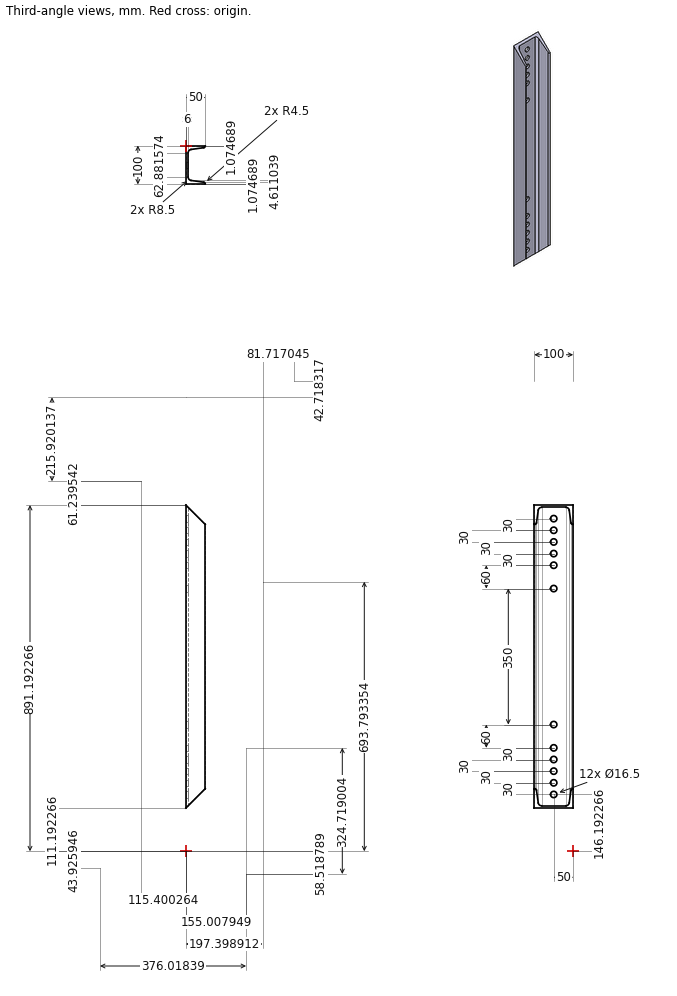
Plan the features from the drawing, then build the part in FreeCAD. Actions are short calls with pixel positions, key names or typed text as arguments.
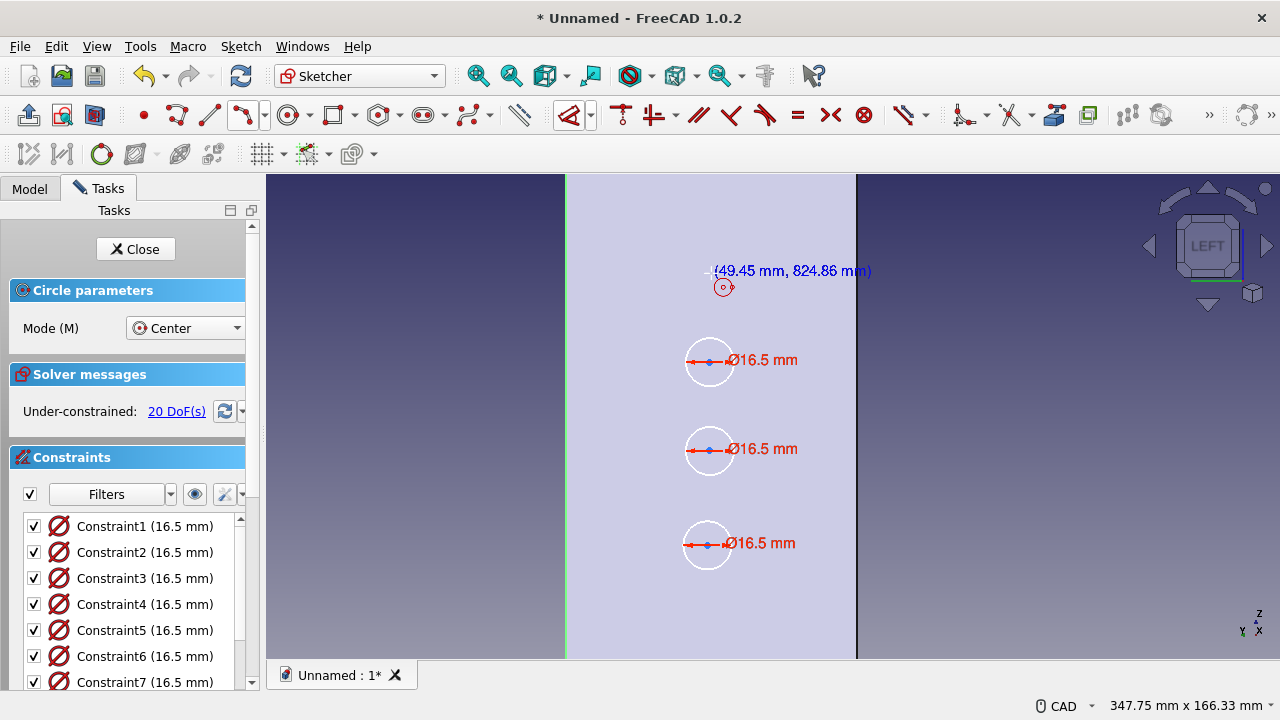
scroll(711, 291, down, 11)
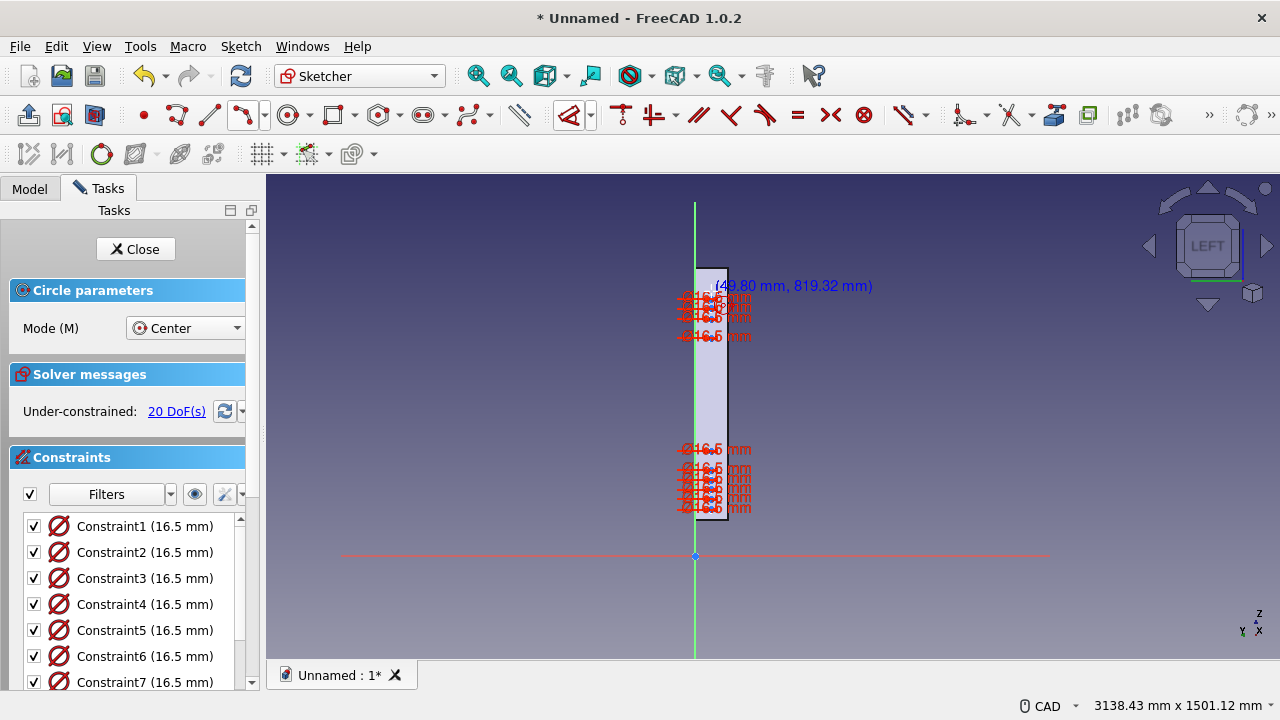
scroll(711, 289, up, 5)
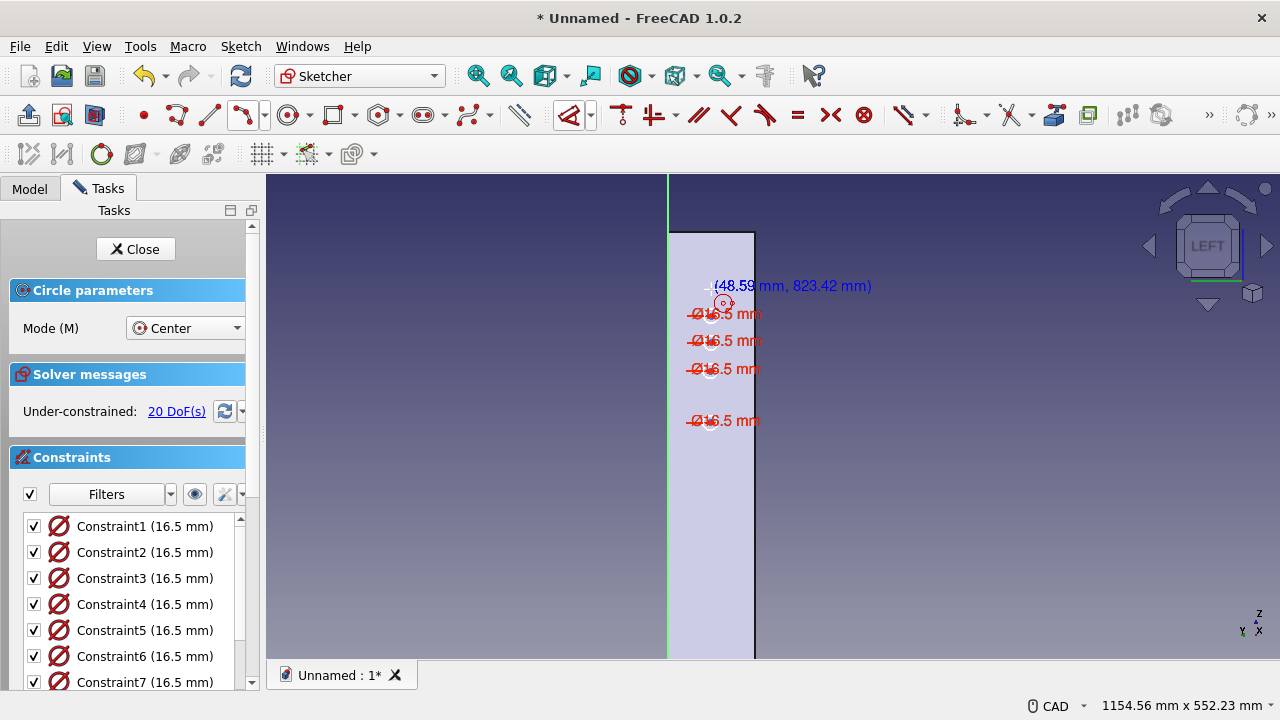
click(711, 289)
move(717, 284)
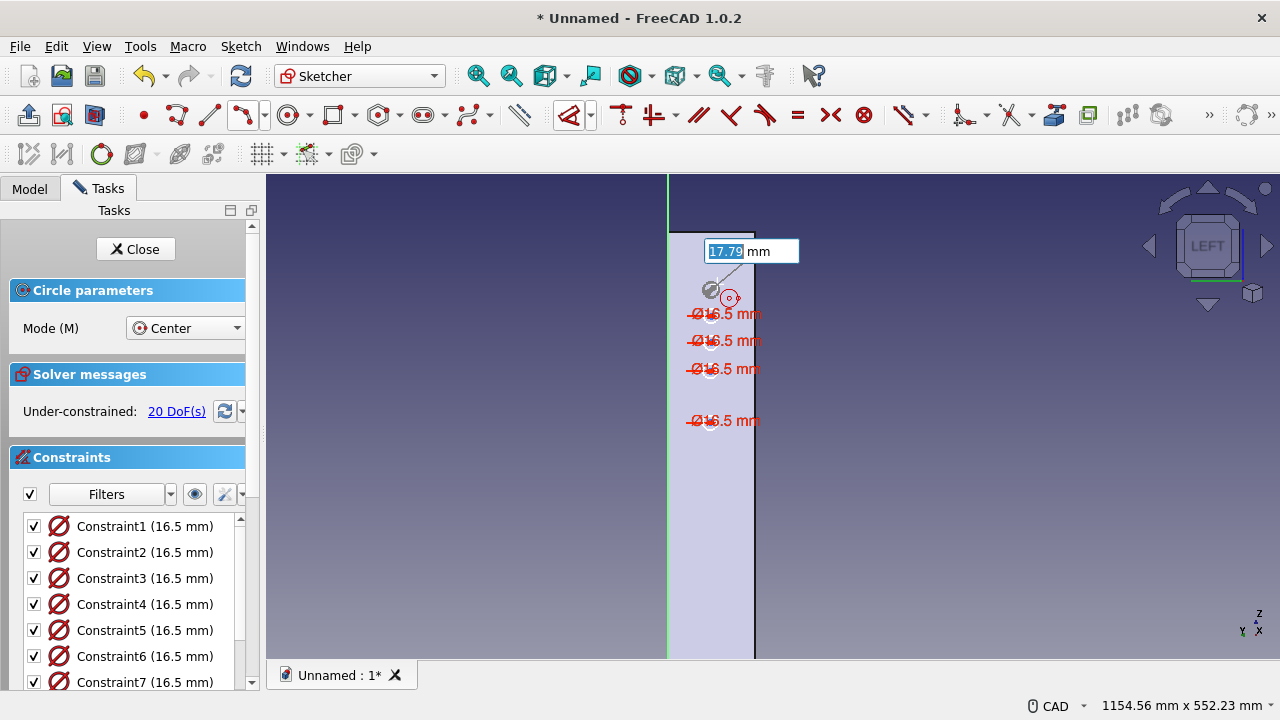
text(16.5)
key(Return)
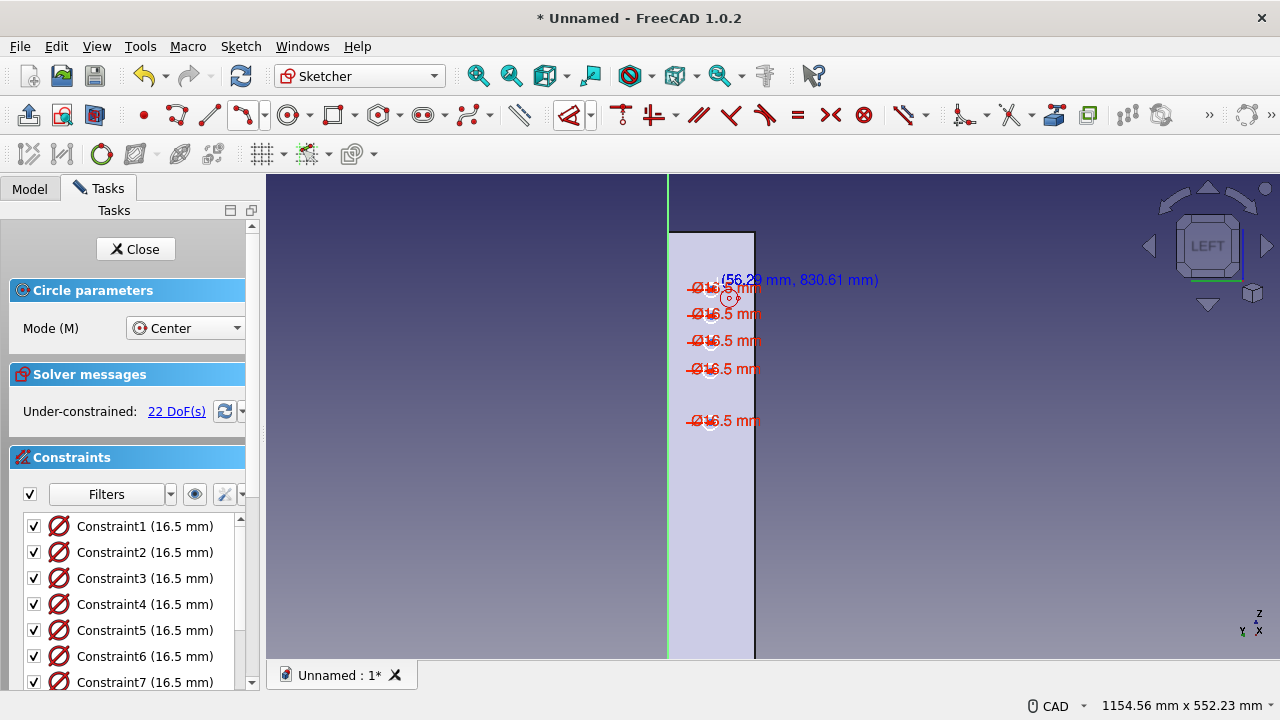
scroll(711, 263, up, 6)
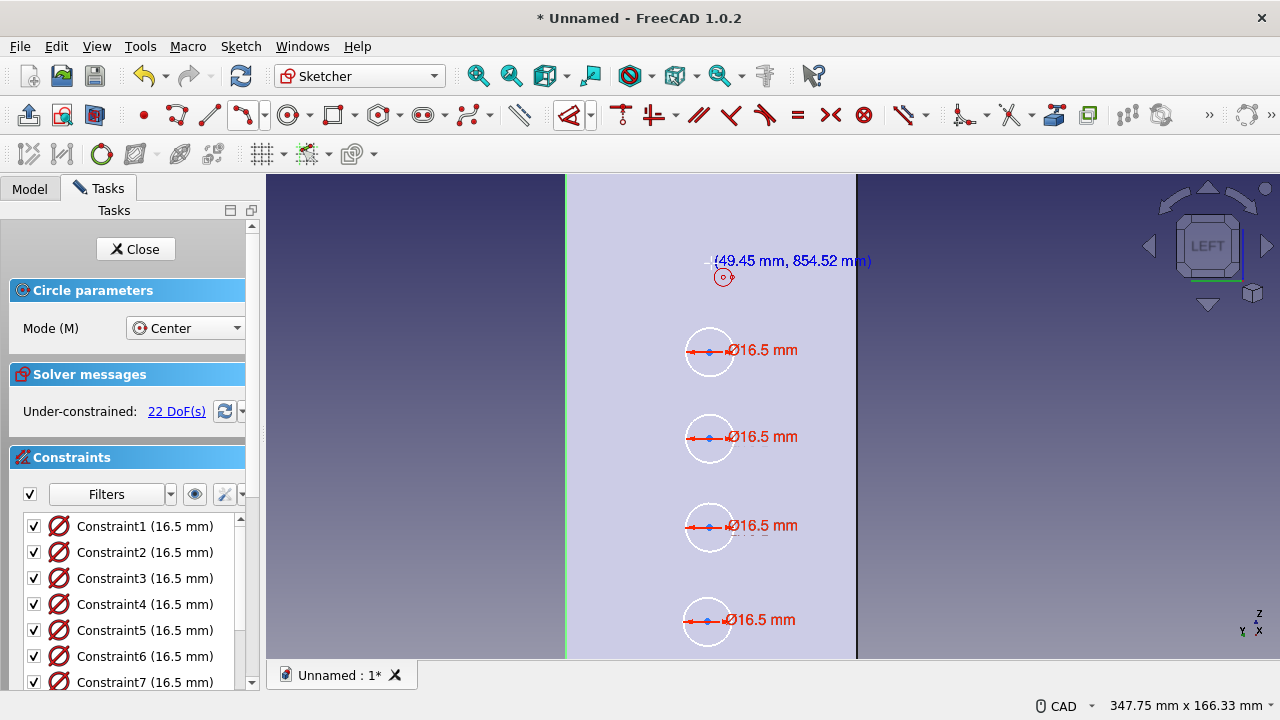
scroll(711, 282, down, 11)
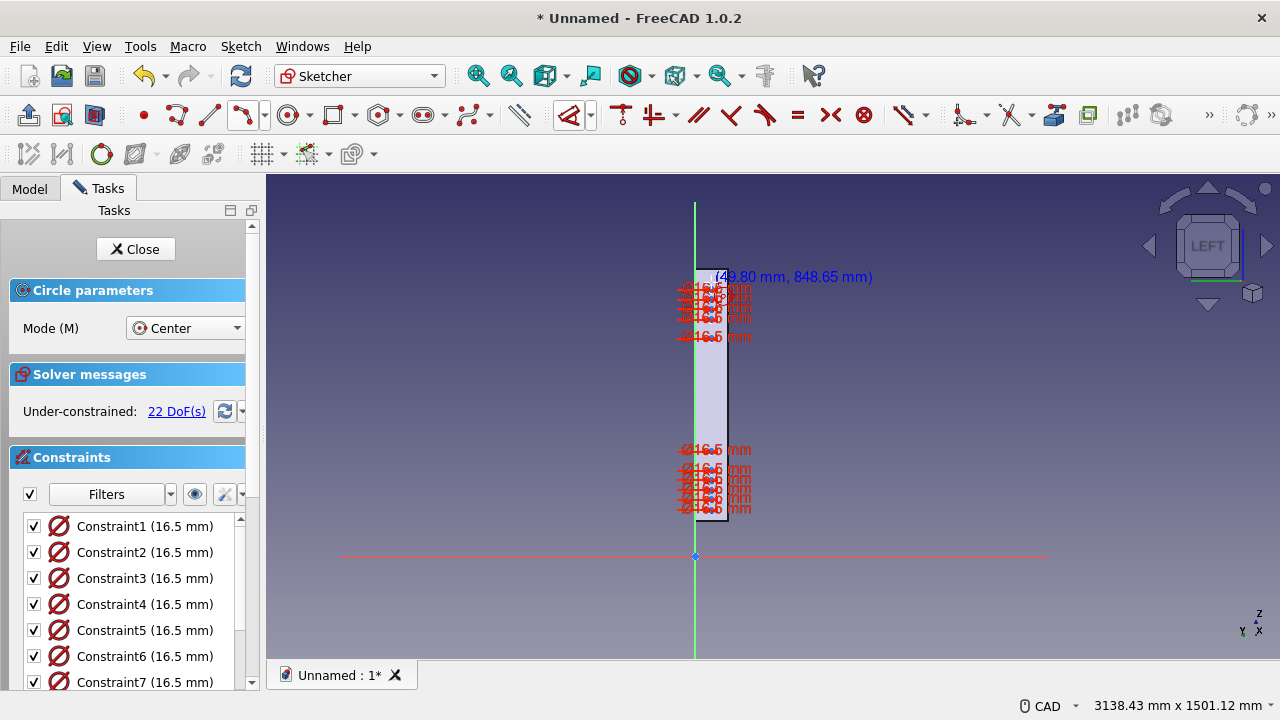
scroll(711, 280, up, 5)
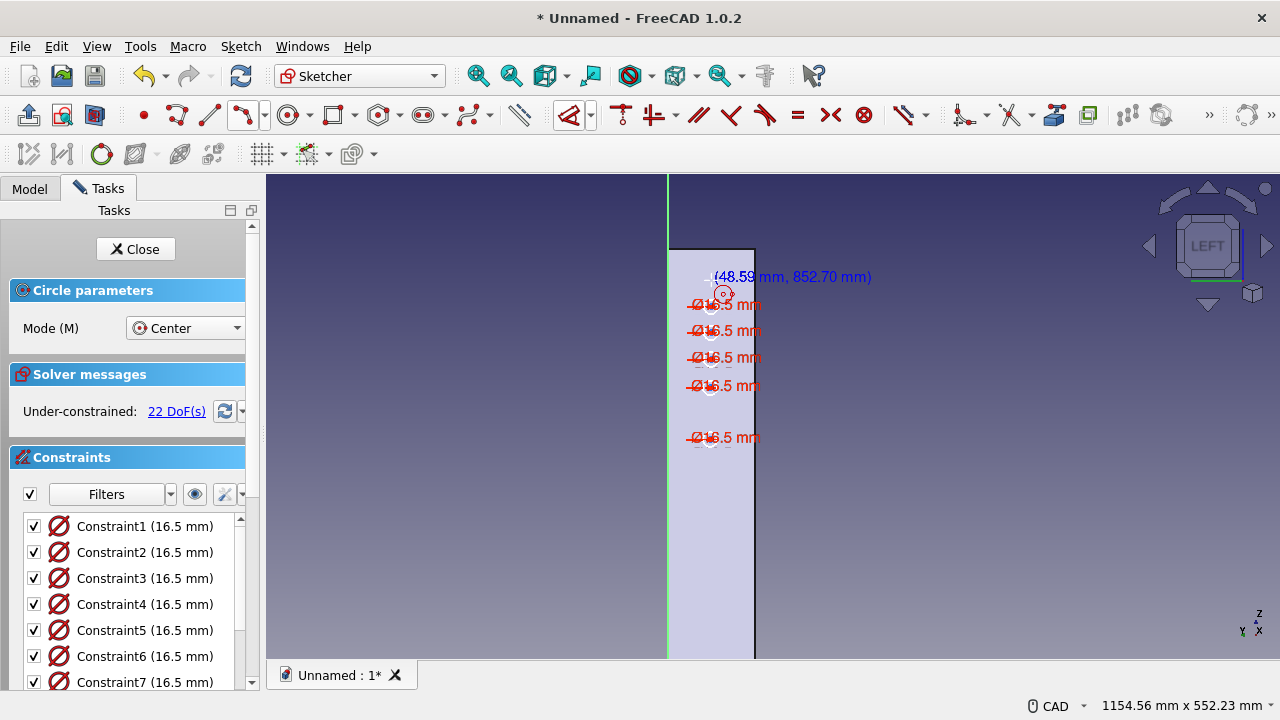
click(711, 279)
move(717, 274)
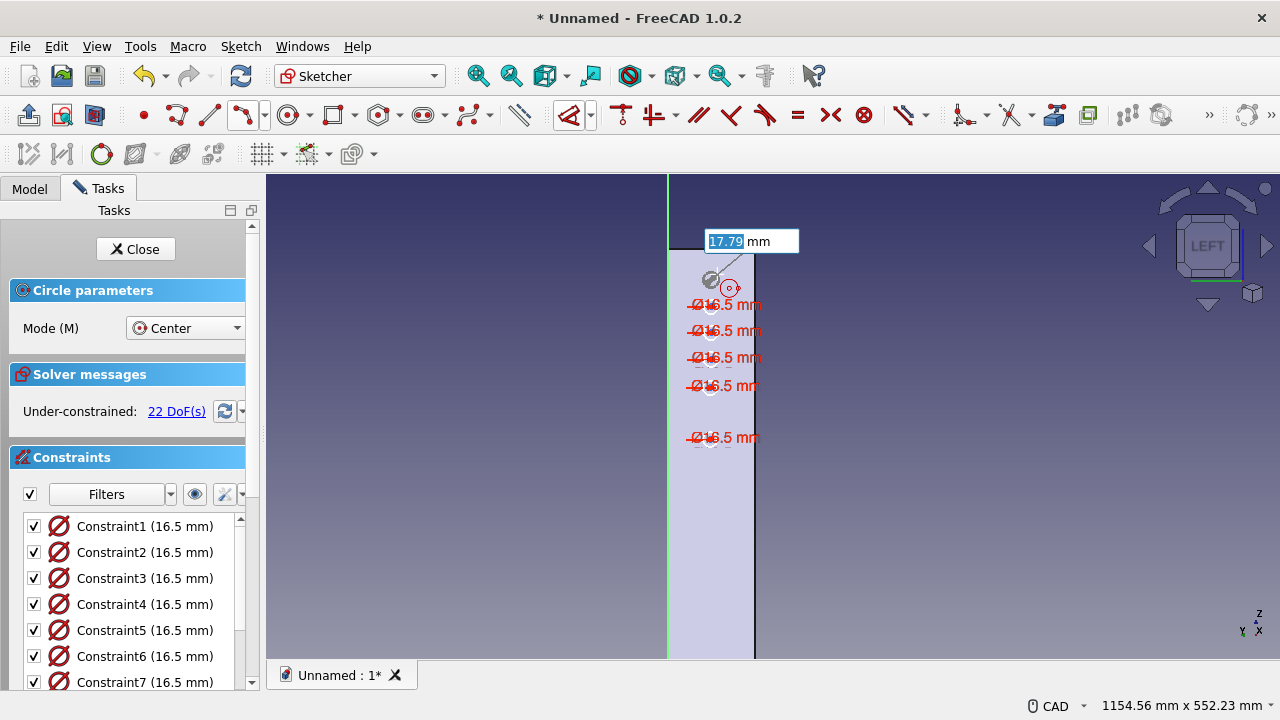
text(16.5)
key(Return)
key(Escape)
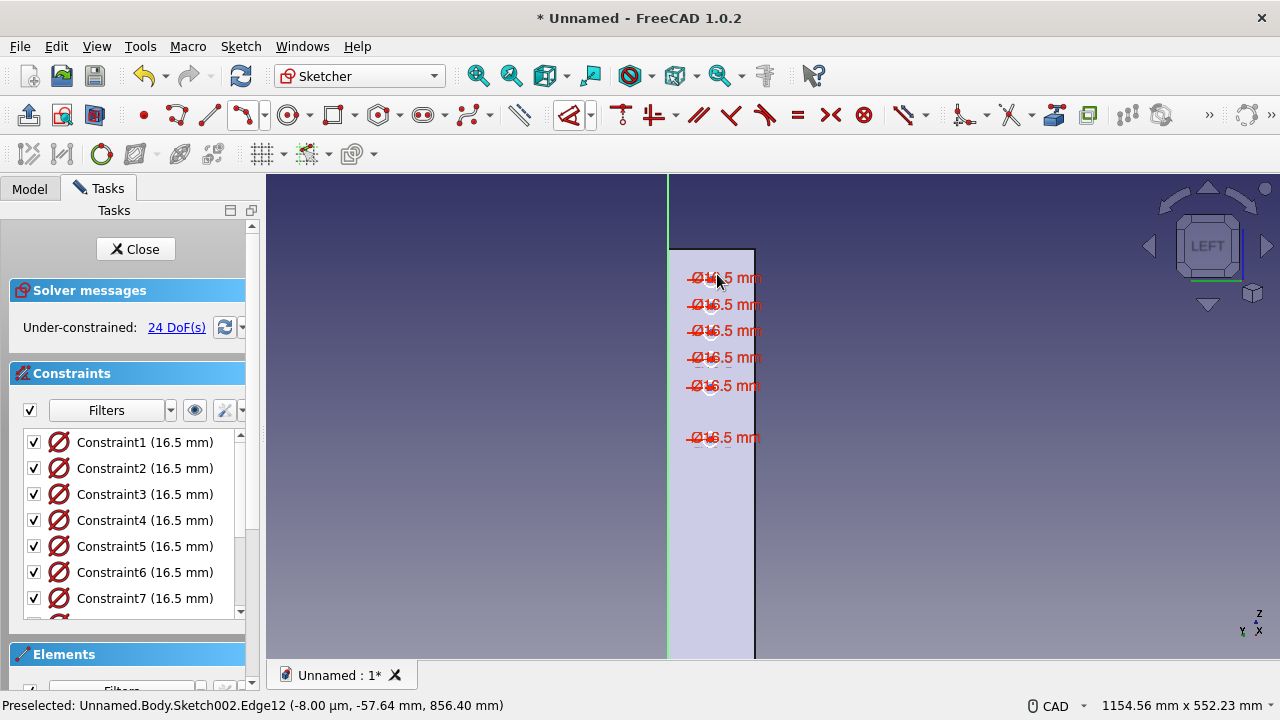
scroll(711, 280, down, 5)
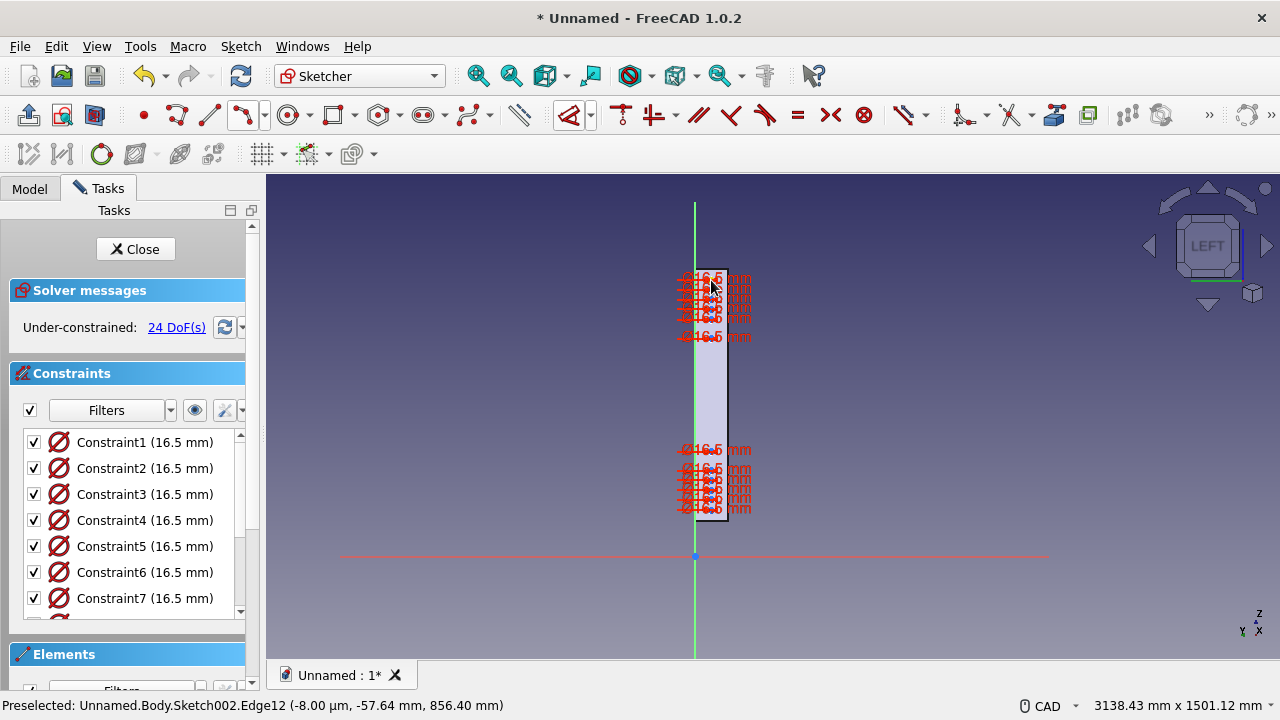
click(711, 510)